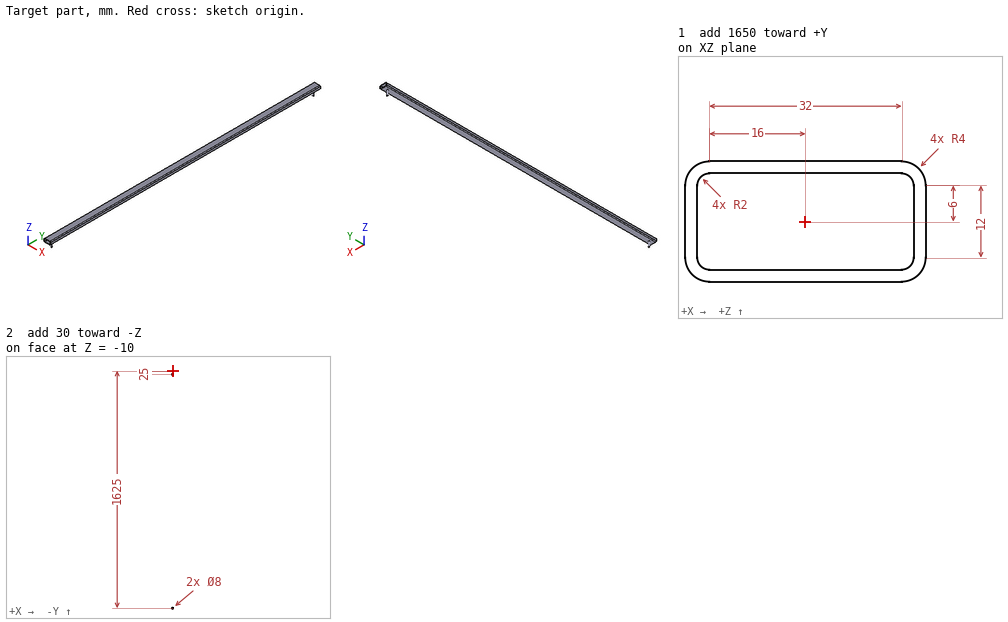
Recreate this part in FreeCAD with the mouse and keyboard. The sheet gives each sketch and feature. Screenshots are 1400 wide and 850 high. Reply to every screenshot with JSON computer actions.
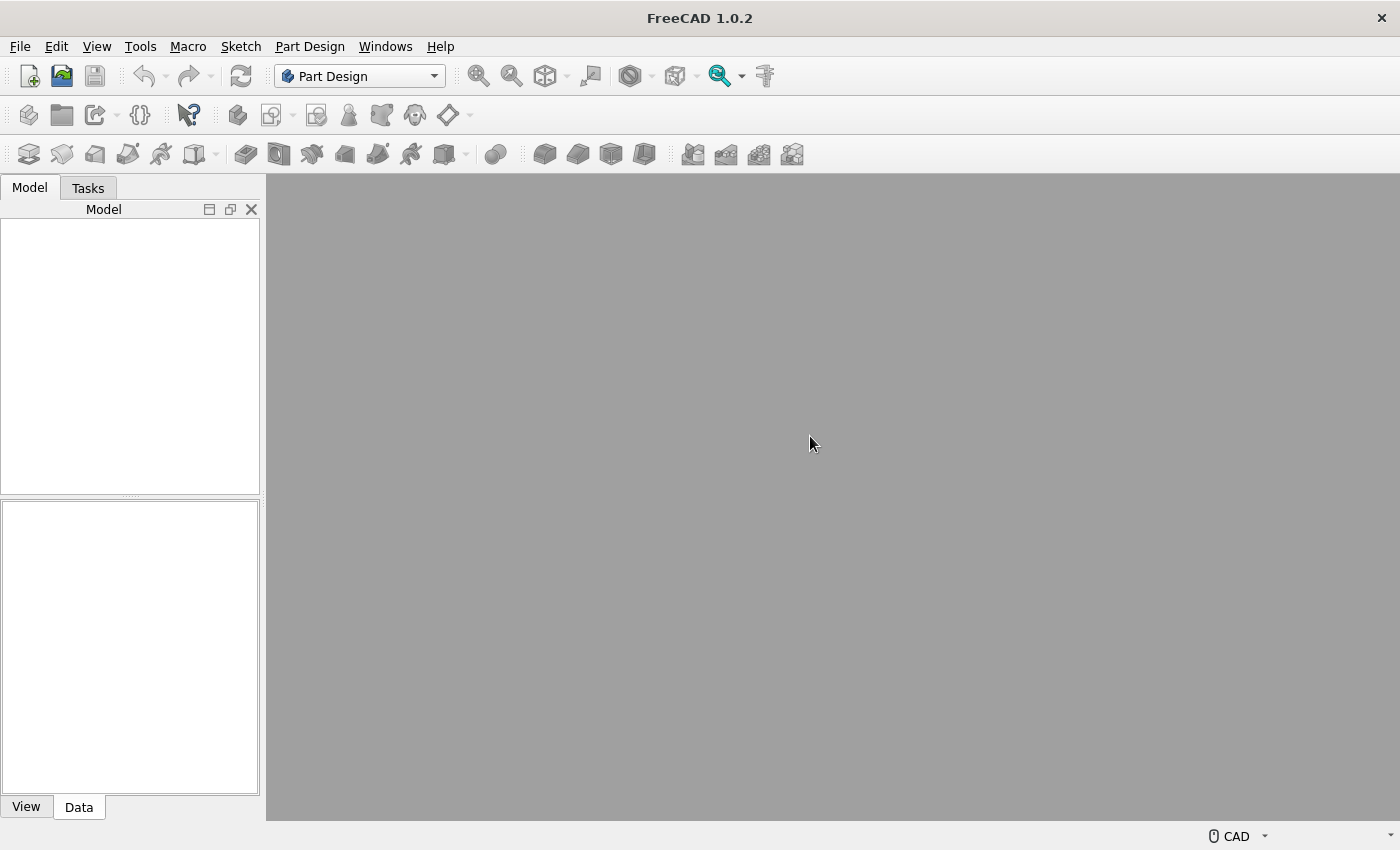
{"action": "left_click", "coordinate": [29, 76]}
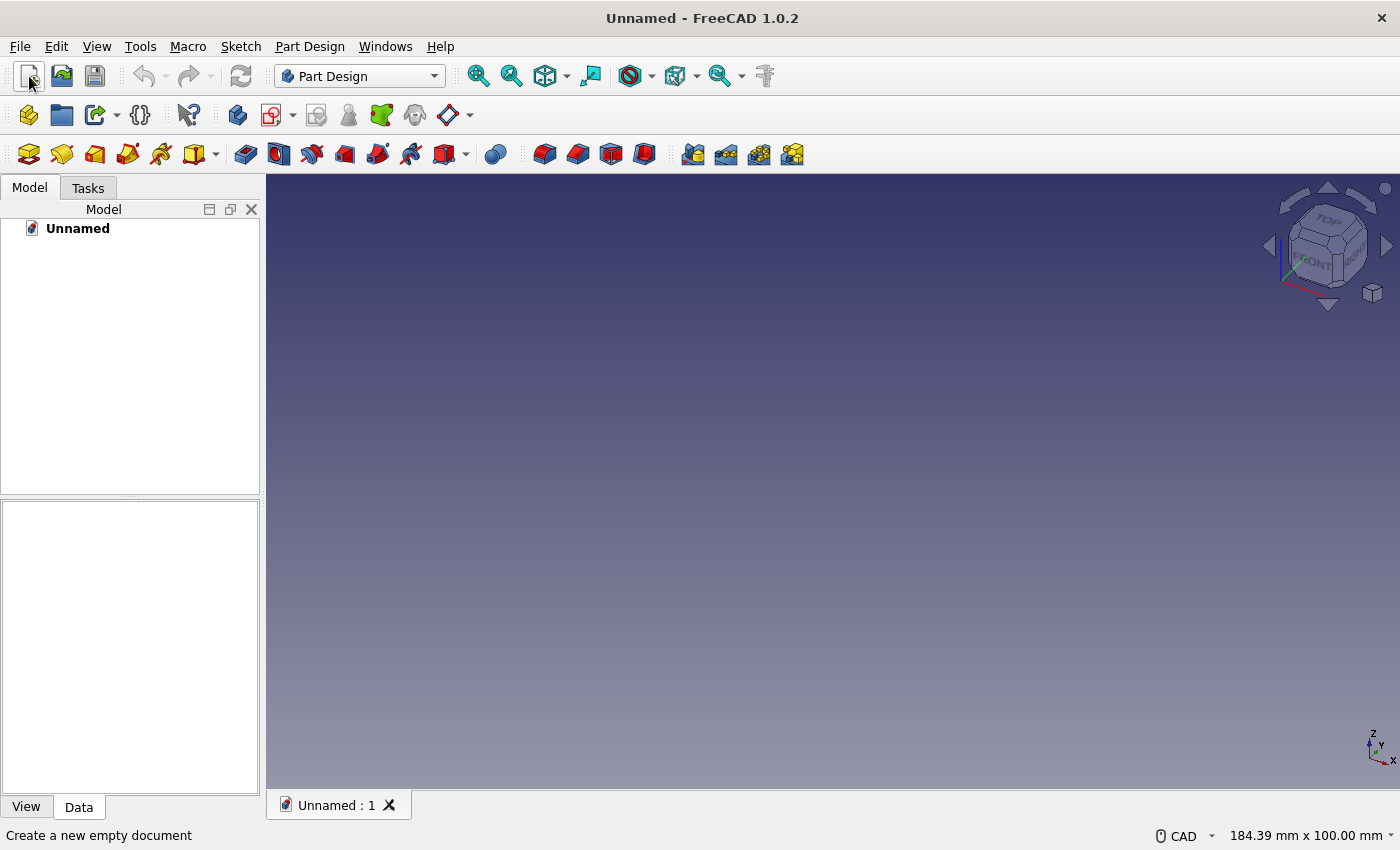
{"action": "left_click", "coordinate": [270, 116]}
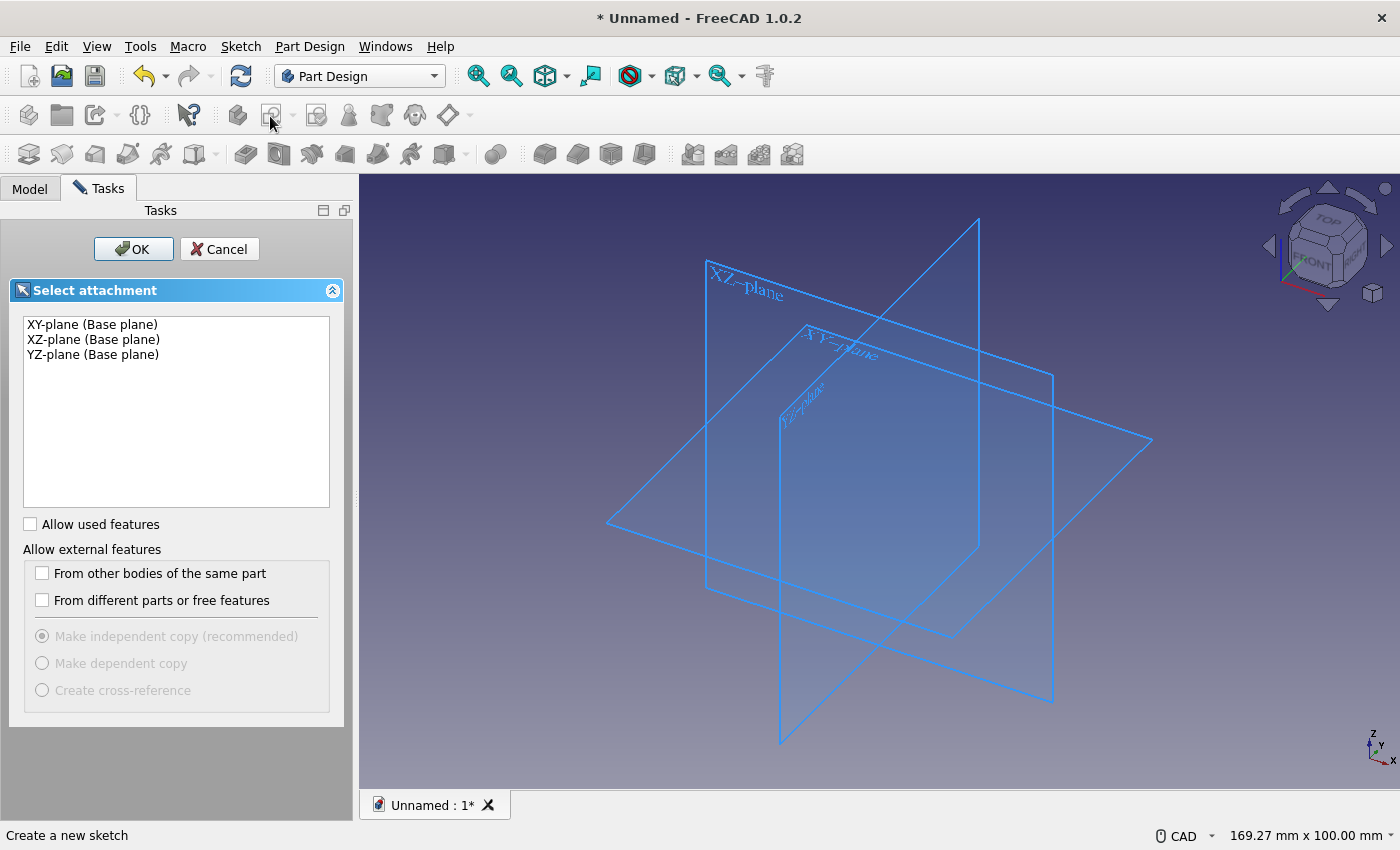
{"action": "left_click", "coordinate": [84, 340]}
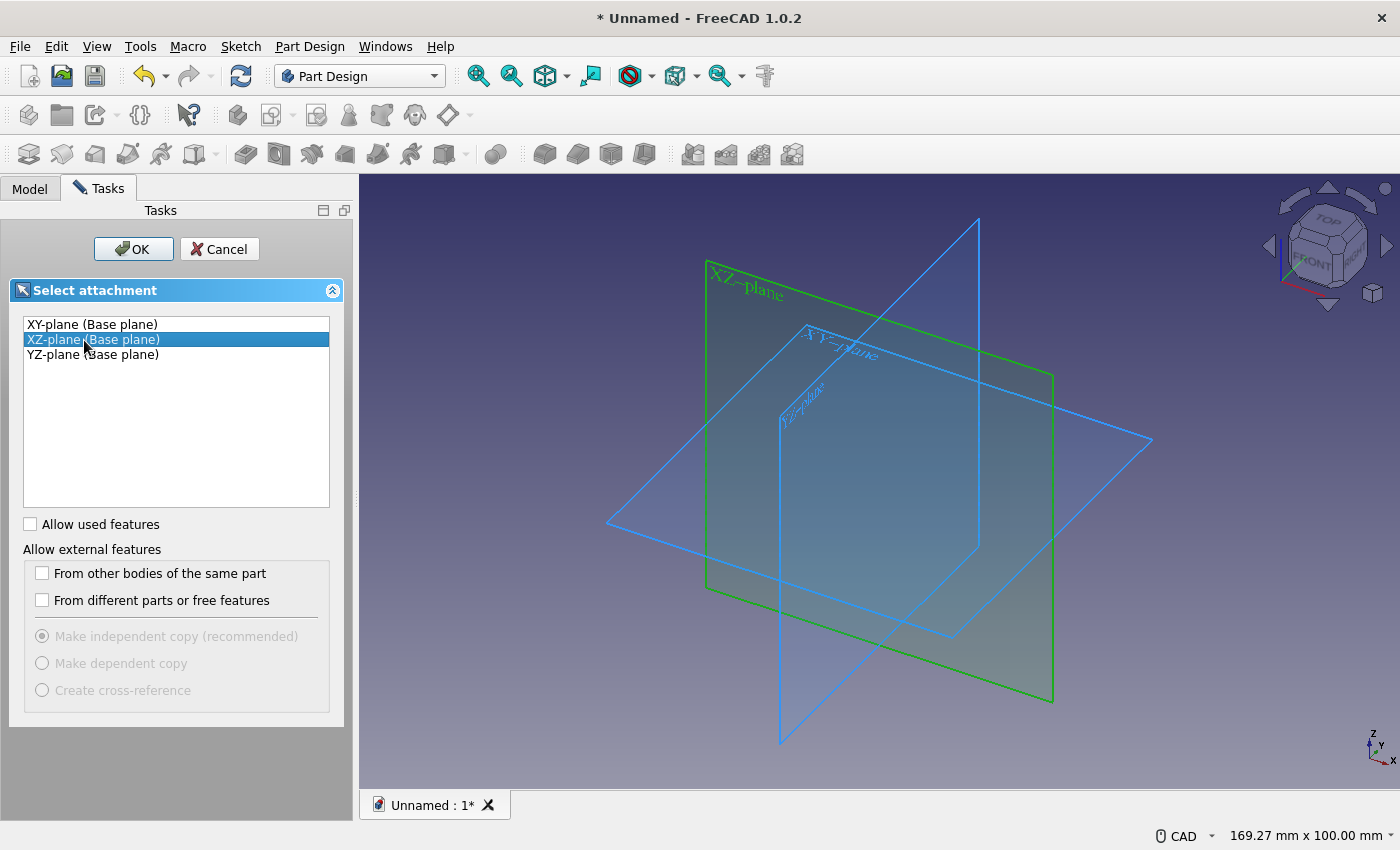
{"action": "left_click", "coordinate": [134, 249]}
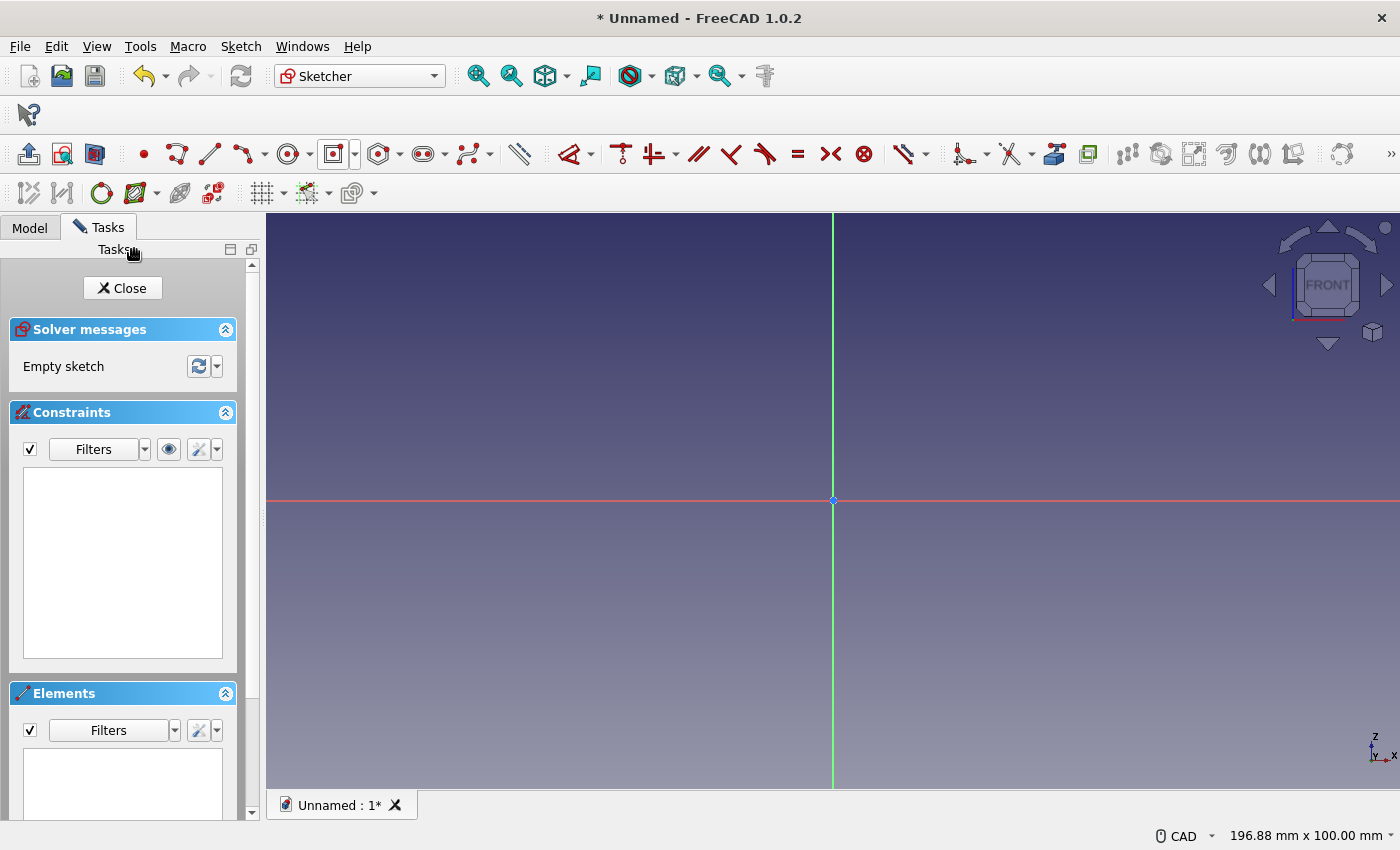
{"action": "scroll", "coordinate": [873, 501], "scroll_direction": "up", "scroll_amount": 5}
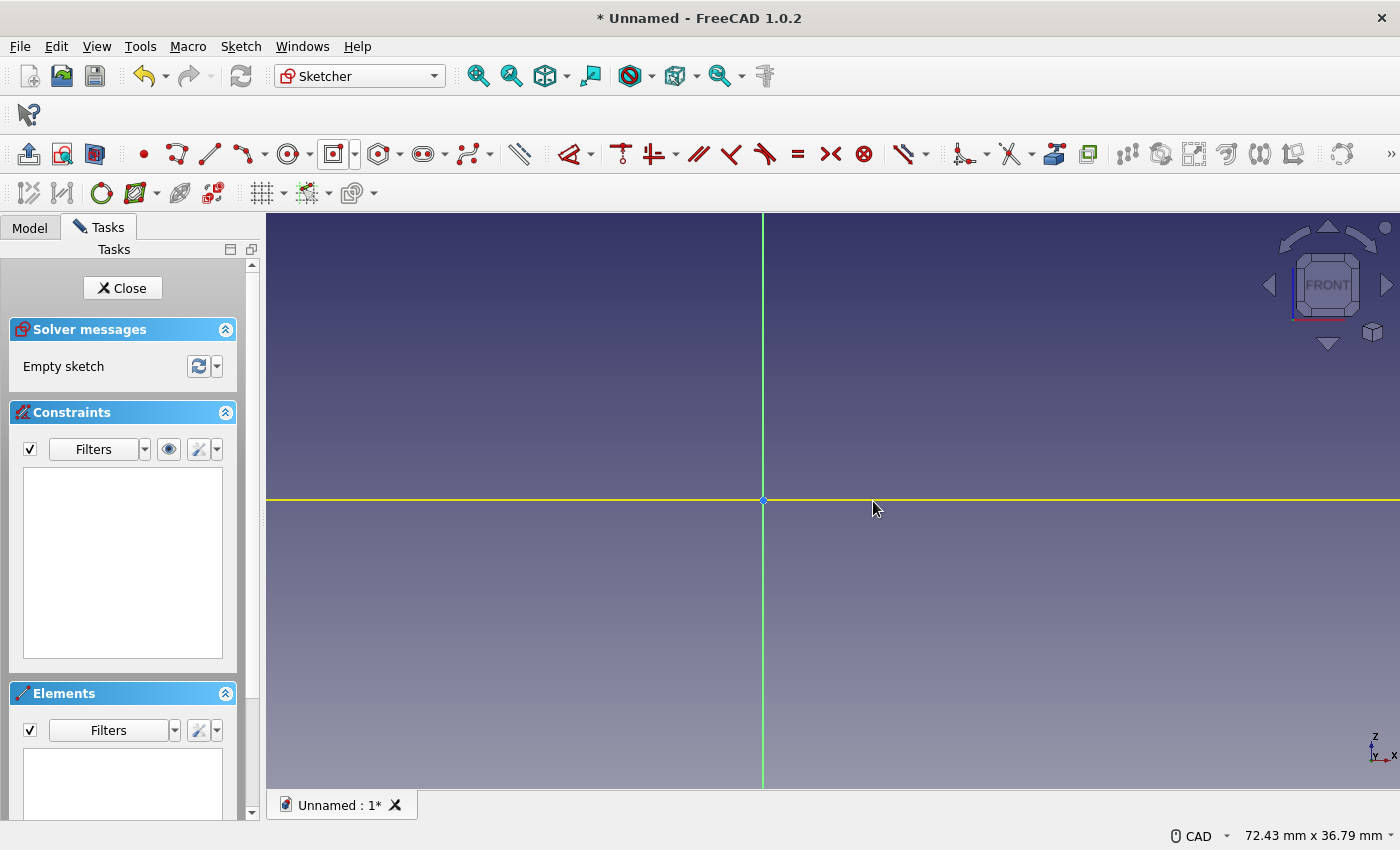
{"action": "left_click", "coordinate": [210, 154]}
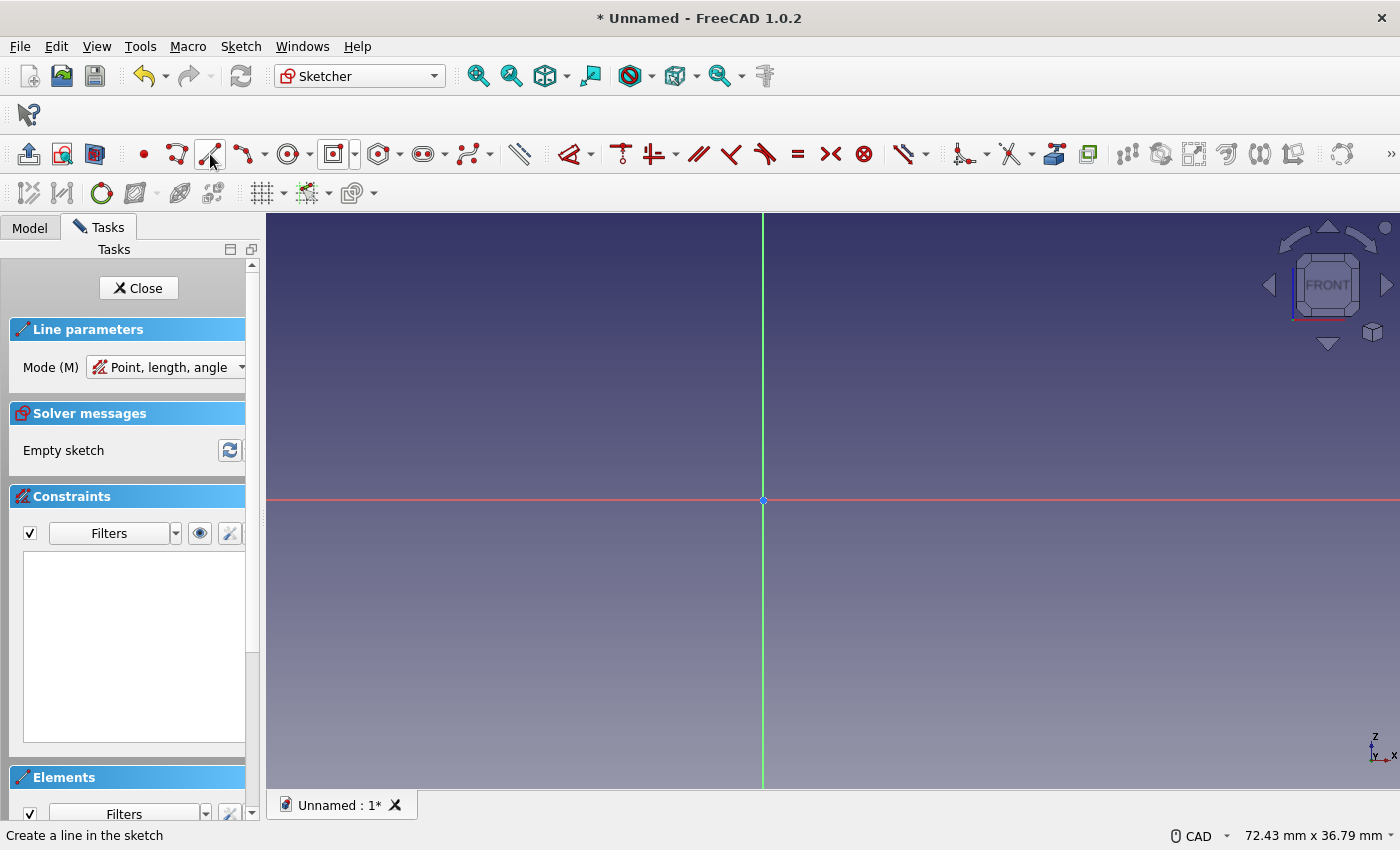
{"action": "left_click", "coordinate": [513, 344]}
{"action": "left_click", "coordinate": [1014, 344]}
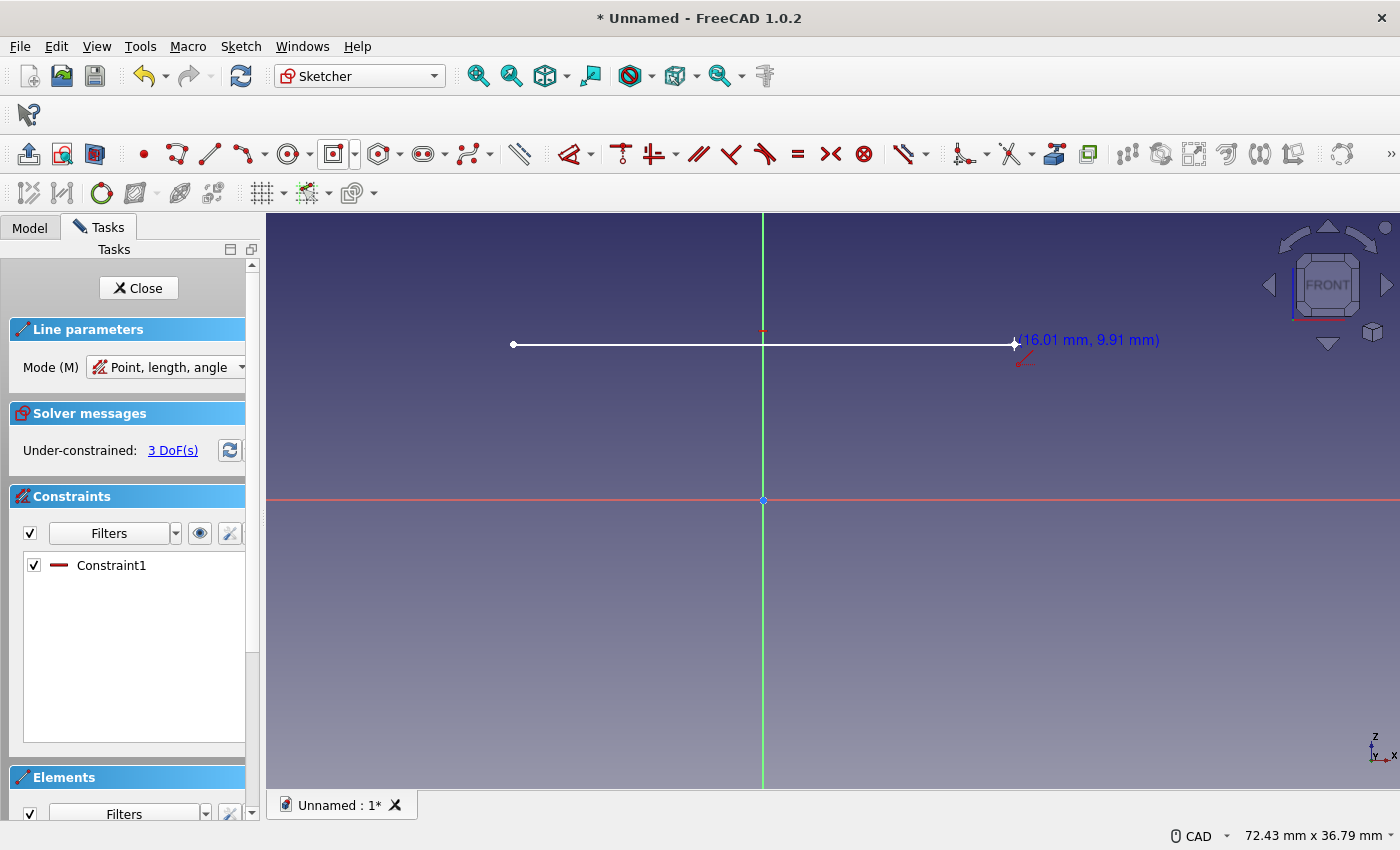
{"action": "left_click", "coordinate": [1076, 406]}
{"action": "left_click", "coordinate": [1076, 594]}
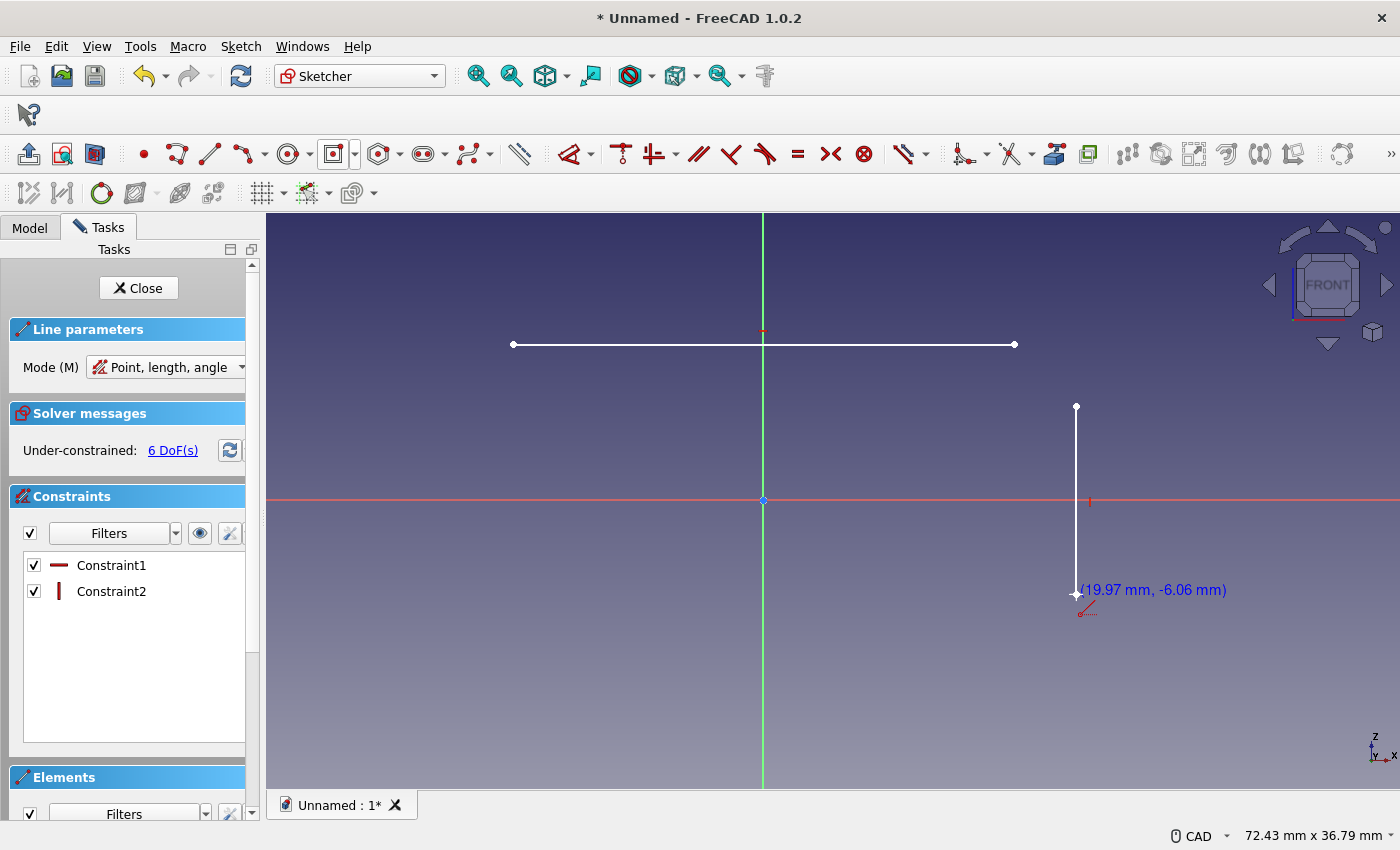
{"action": "left_click", "coordinate": [1014, 657]}
{"action": "left_click", "coordinate": [513, 657]}